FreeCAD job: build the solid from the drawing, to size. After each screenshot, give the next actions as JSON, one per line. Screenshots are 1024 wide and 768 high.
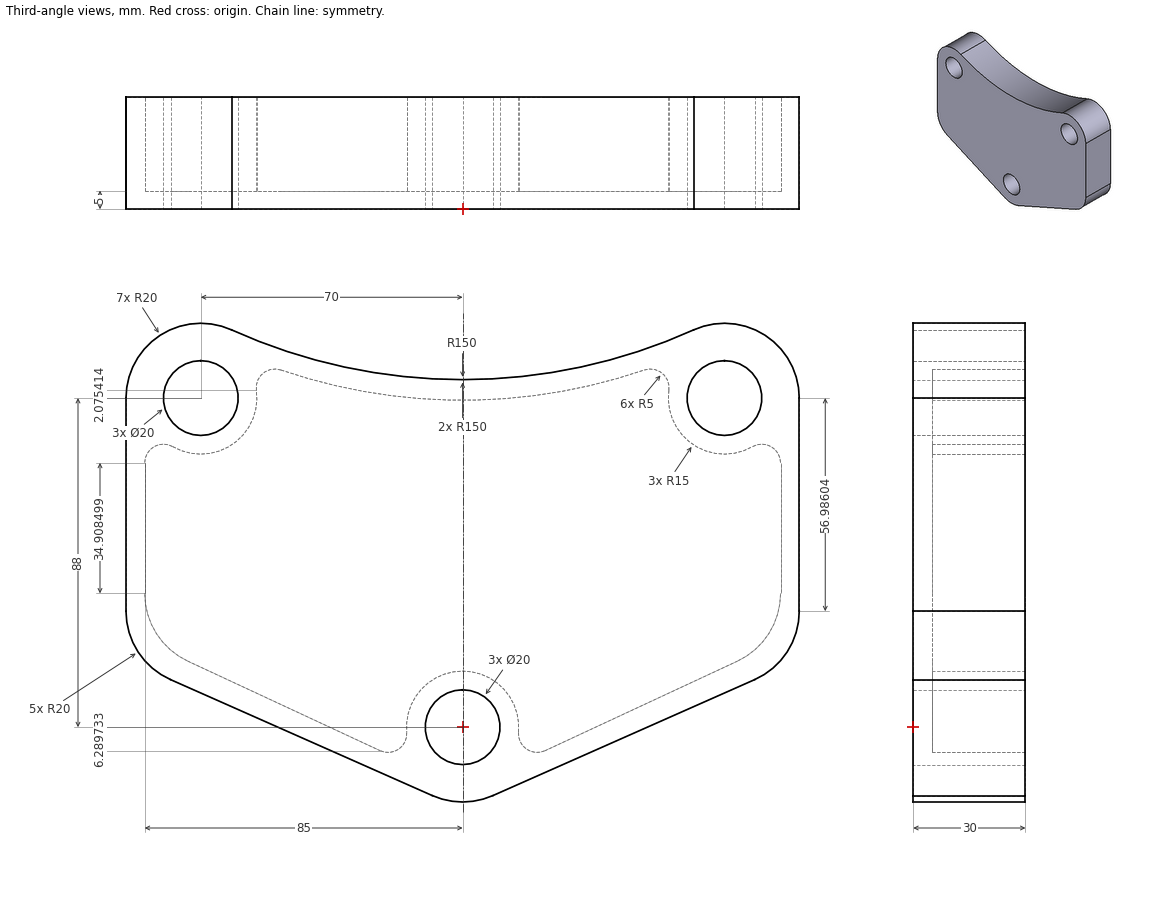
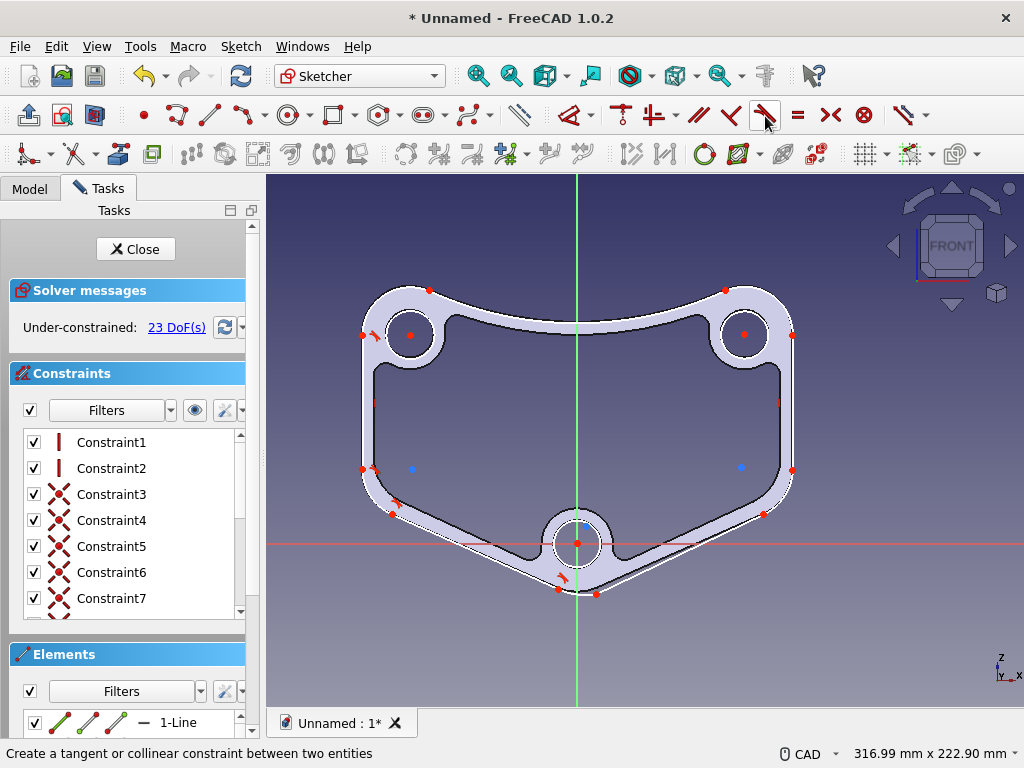
{"action": "left_click", "coordinate": [646, 570]}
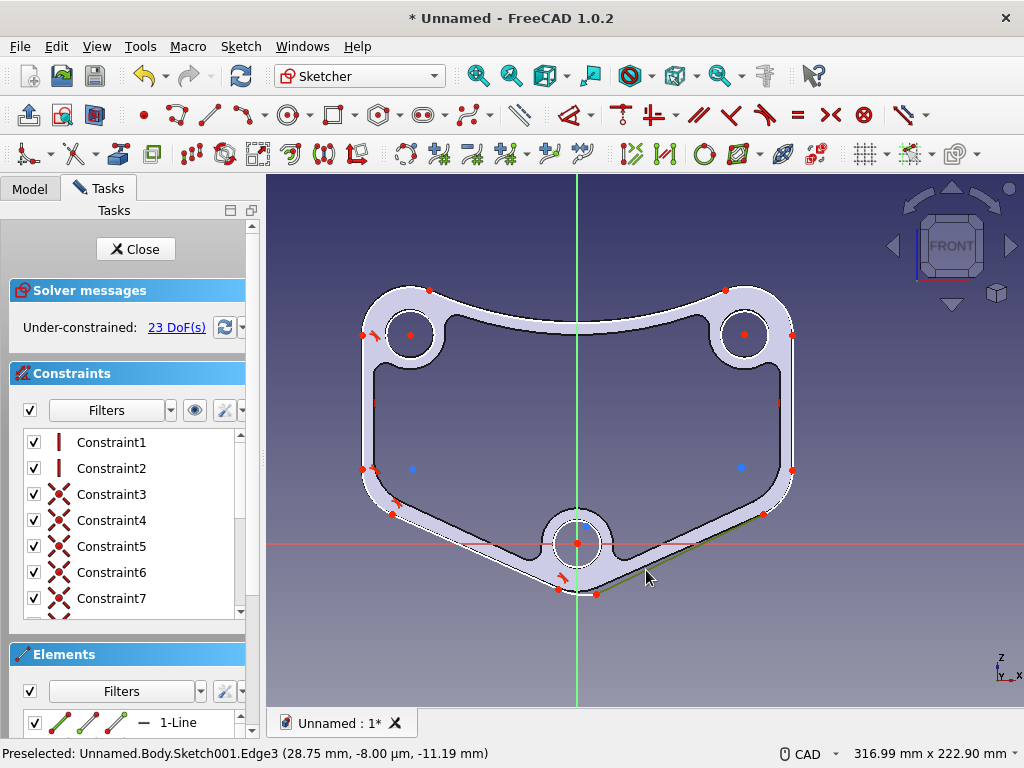
{"action": "left_click", "coordinate": [577, 595]}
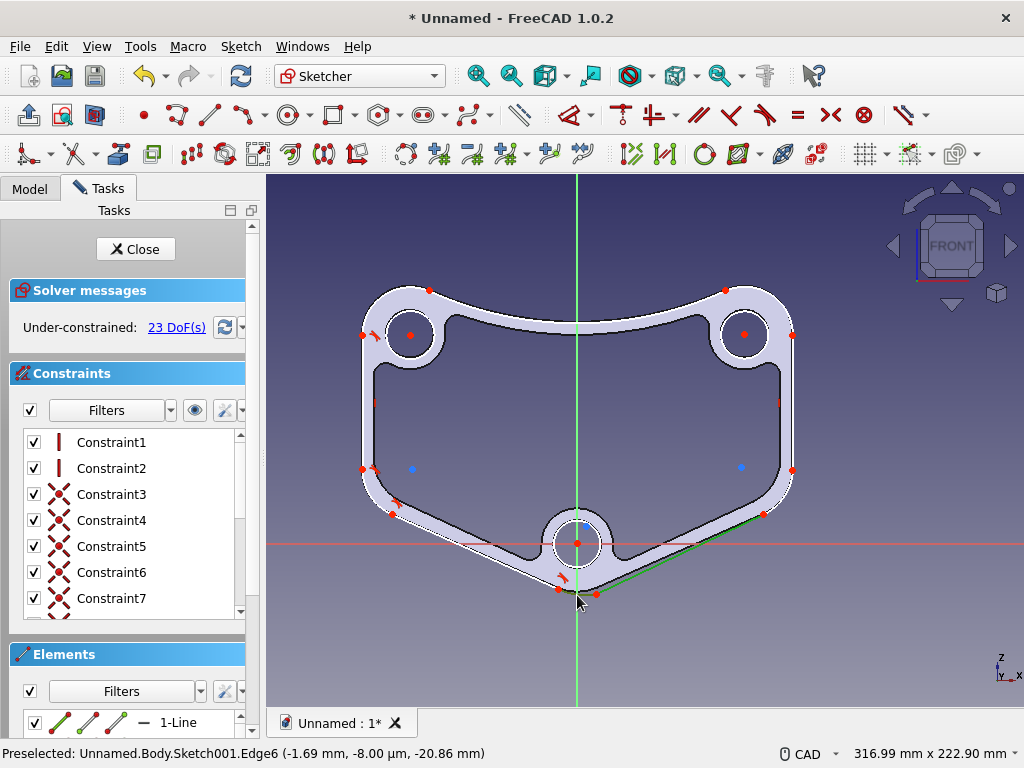
{"action": "left_click", "coordinate": [765, 116]}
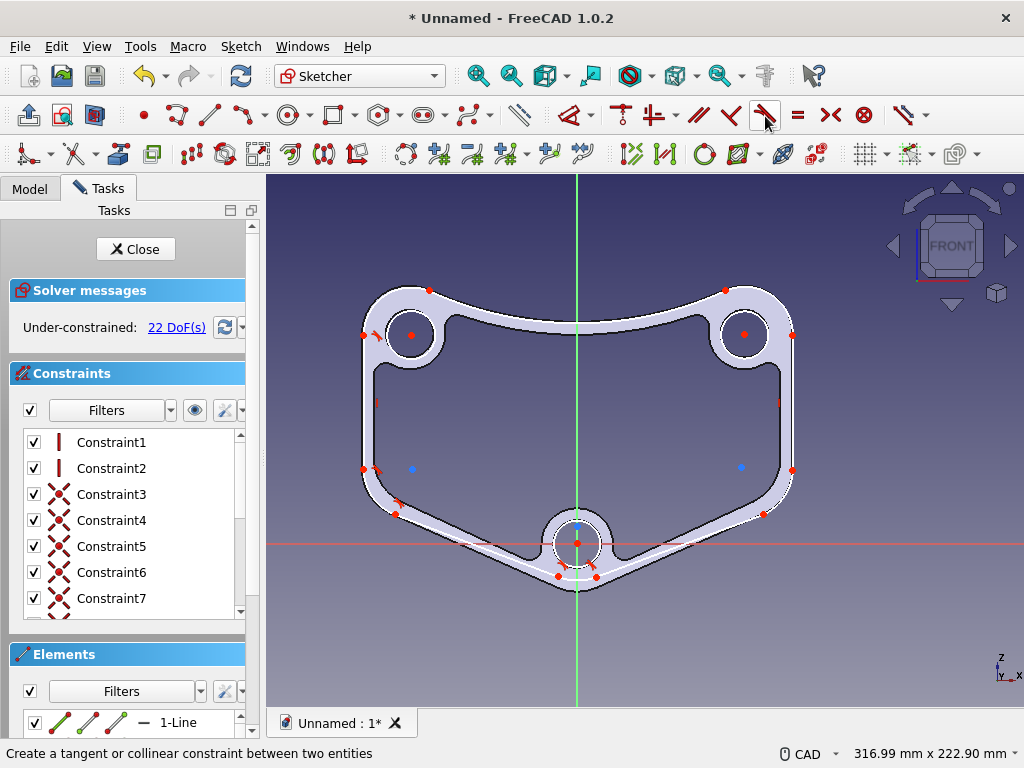
{"action": "left_click", "coordinate": [646, 558]}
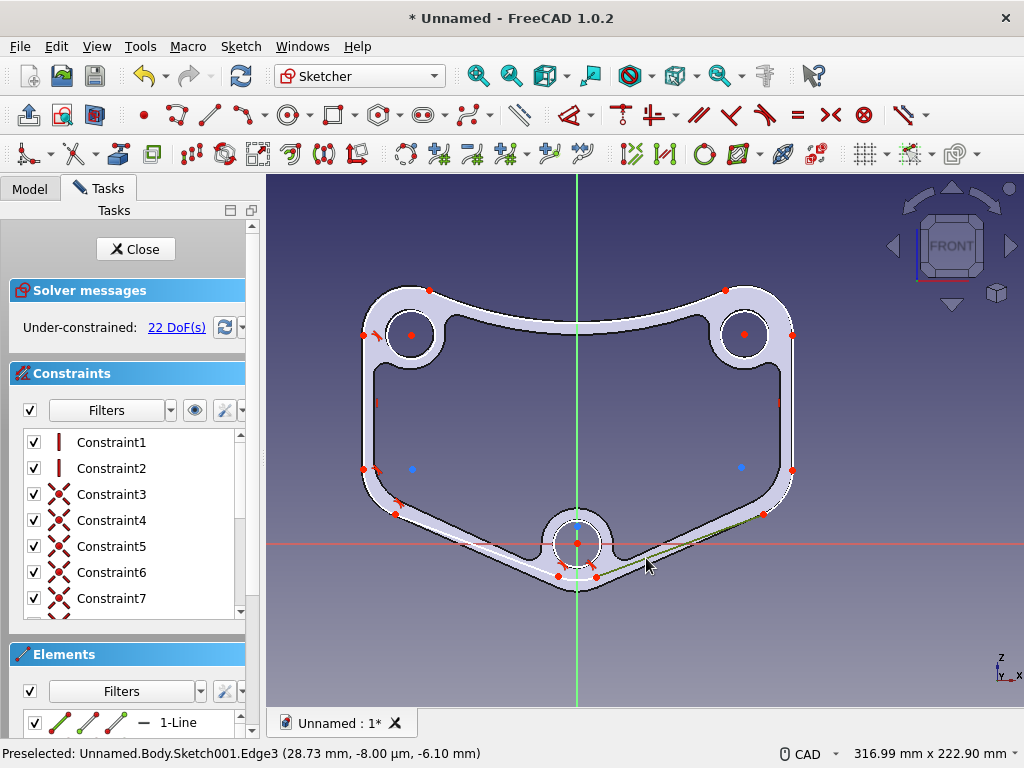
{"action": "left_click", "coordinate": [777, 505]}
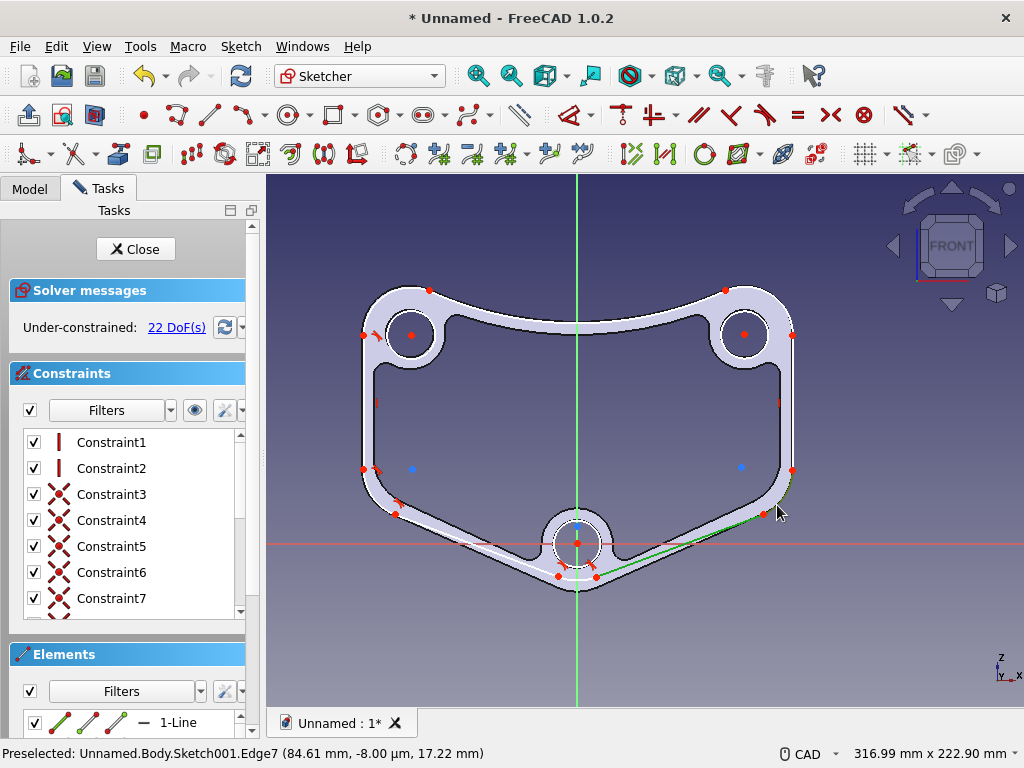
{"action": "left_click", "coordinate": [765, 116]}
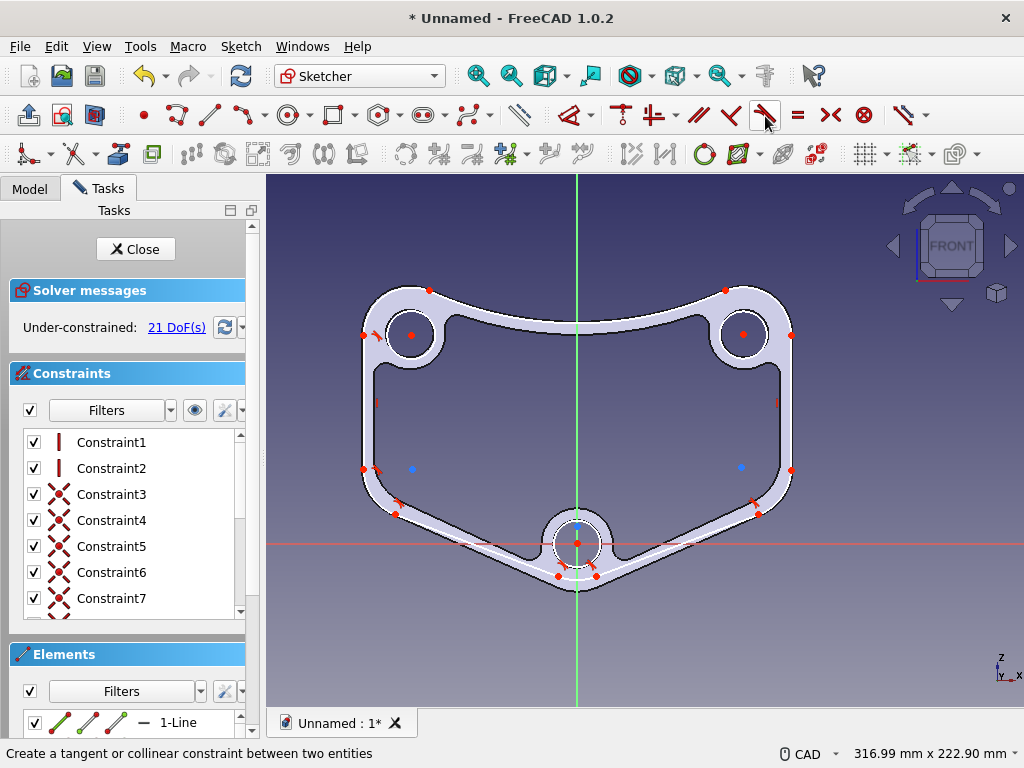
{"action": "left_click", "coordinate": [791, 430]}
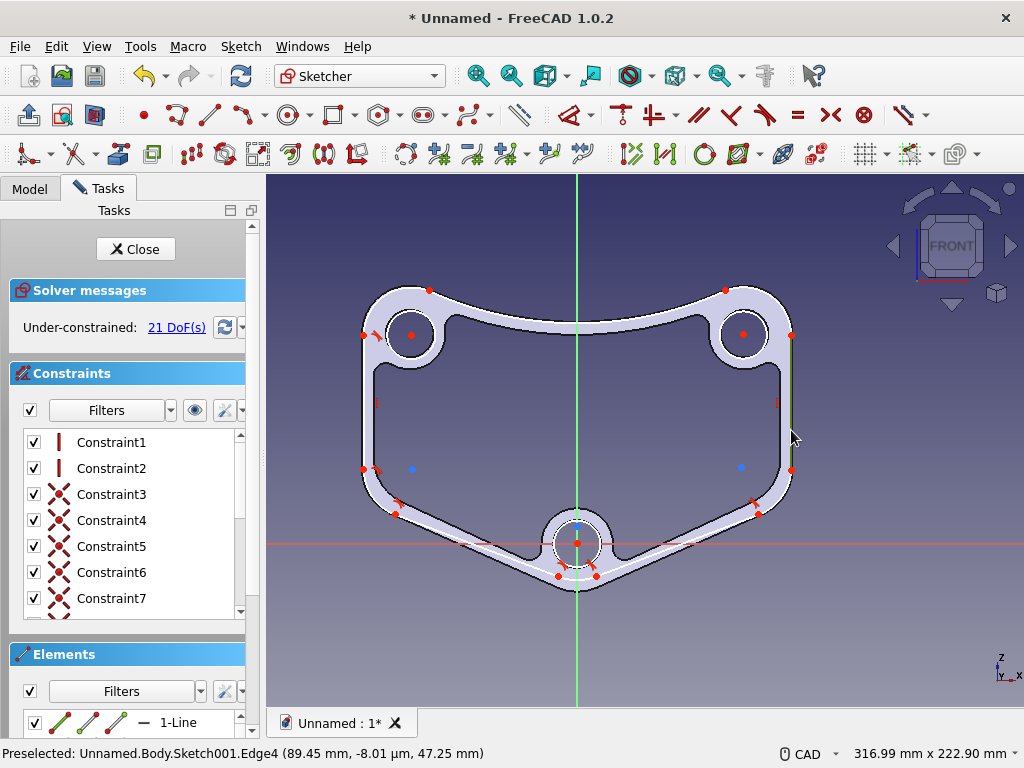
{"action": "left_click", "coordinate": [774, 506]}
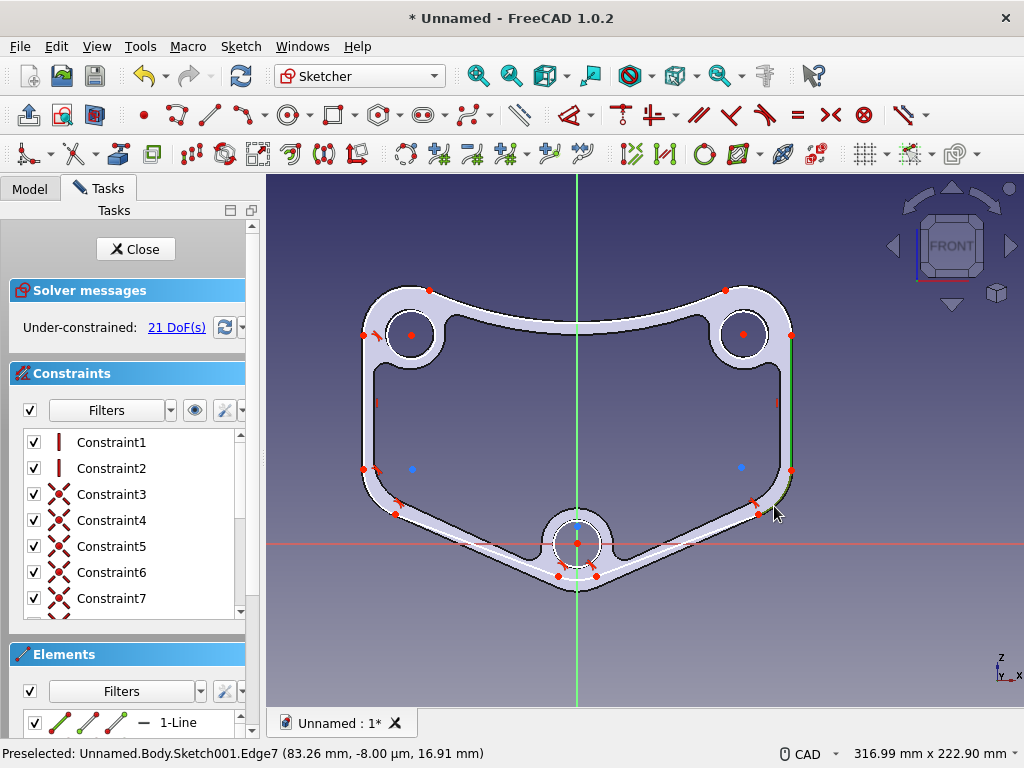
{"action": "left_click", "coordinate": [765, 116]}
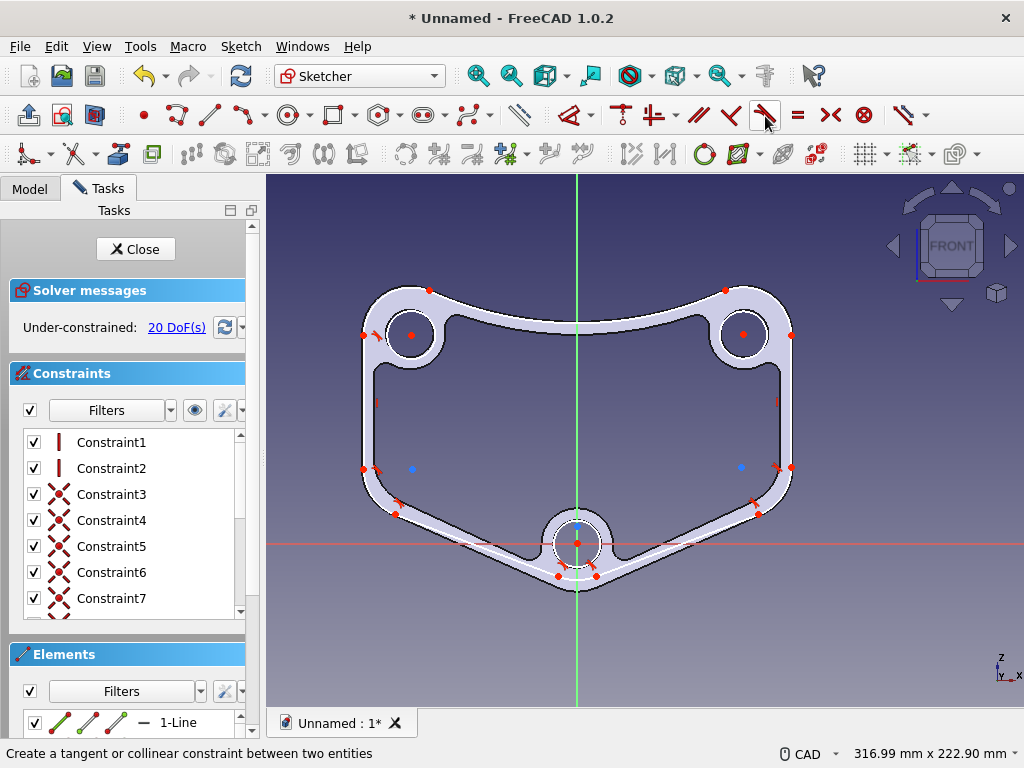
{"action": "left_click", "coordinate": [791, 428]}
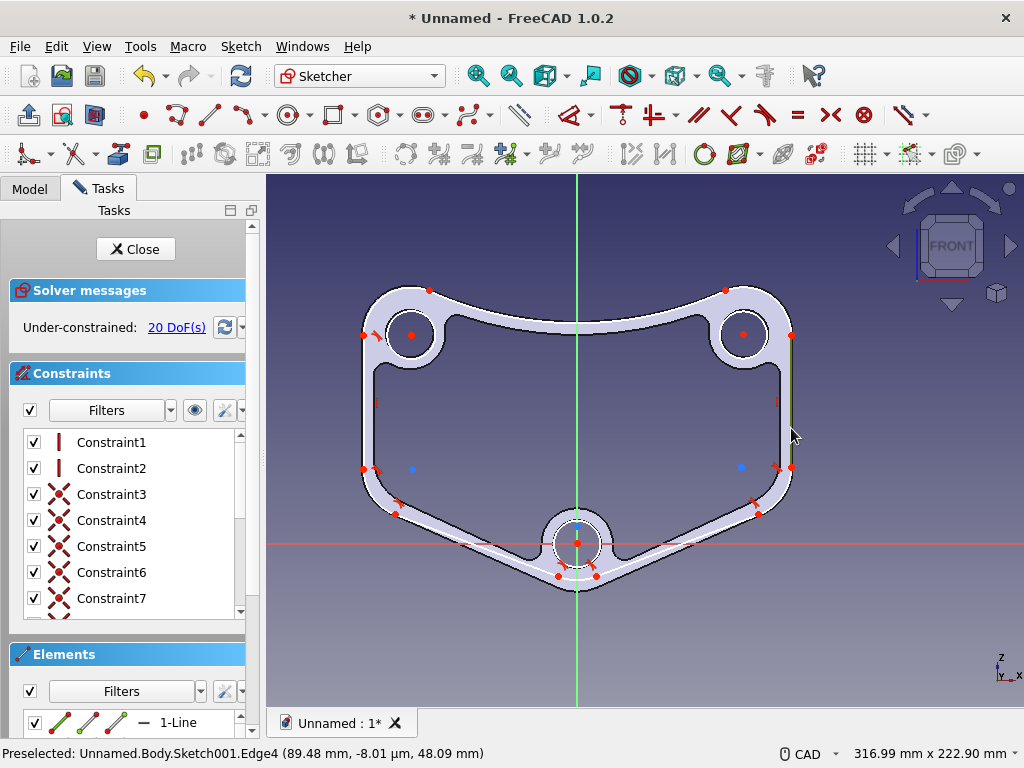
{"action": "left_click", "coordinate": [783, 309]}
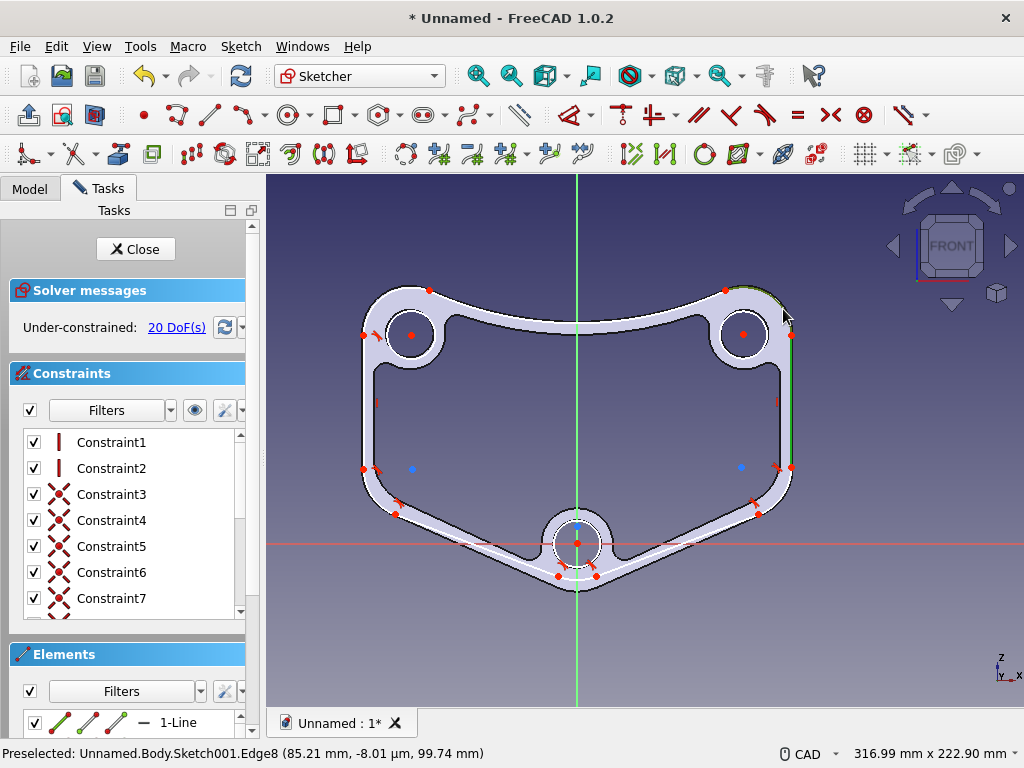
{"action": "key", "text": "t"}